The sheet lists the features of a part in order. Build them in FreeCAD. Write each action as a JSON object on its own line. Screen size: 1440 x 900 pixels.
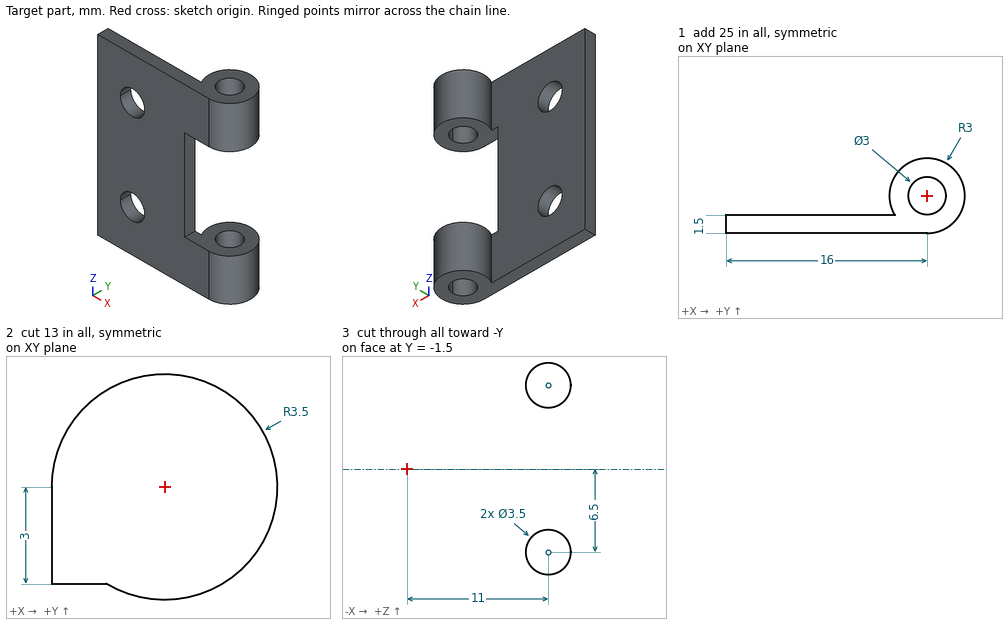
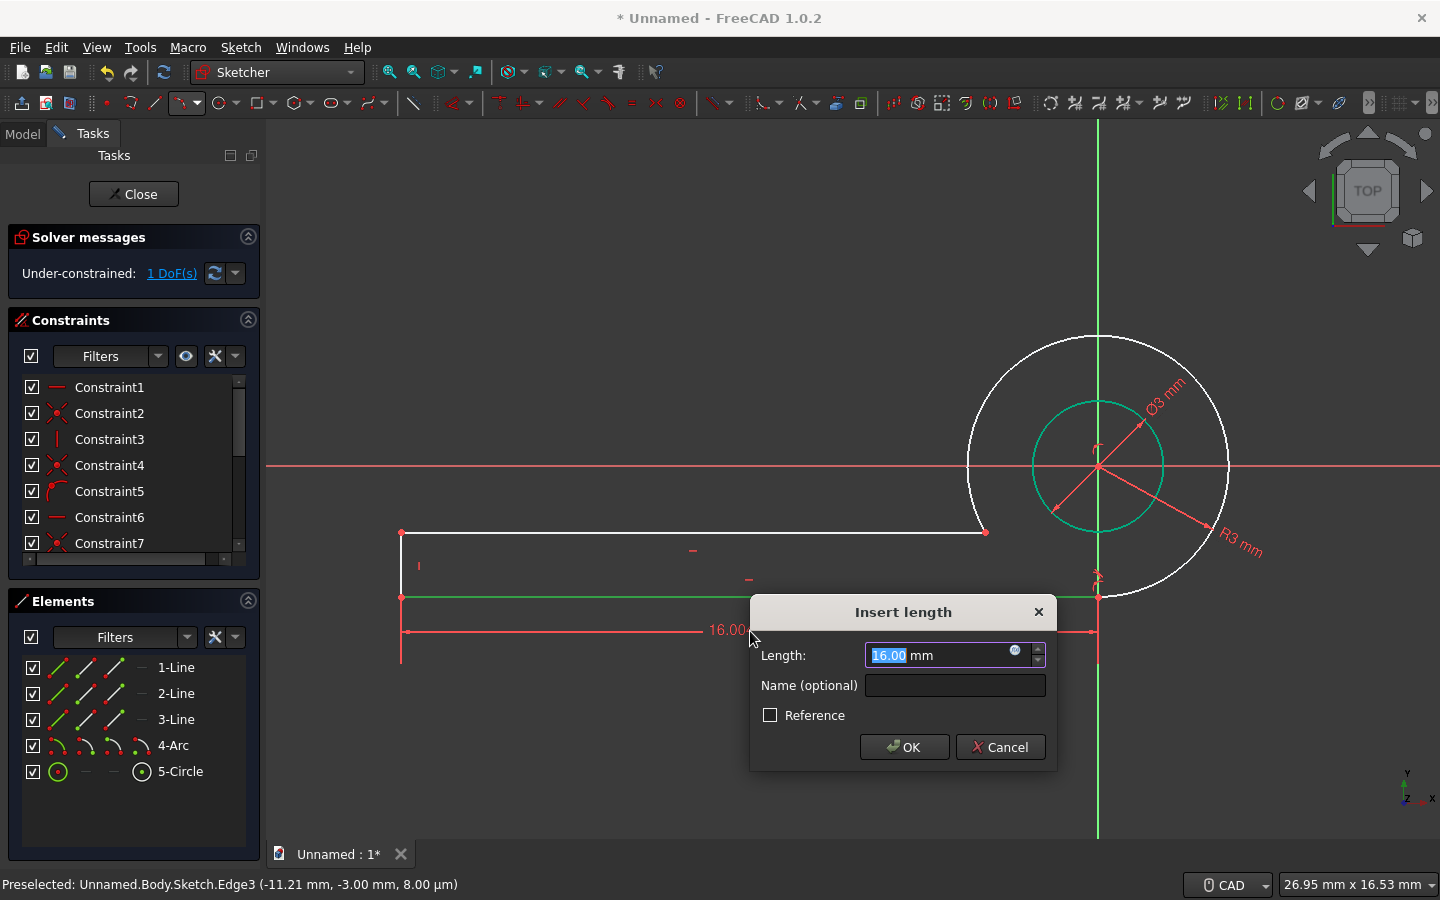
{"action": "type", "text": "16"}
{"action": "key", "text": "Return"}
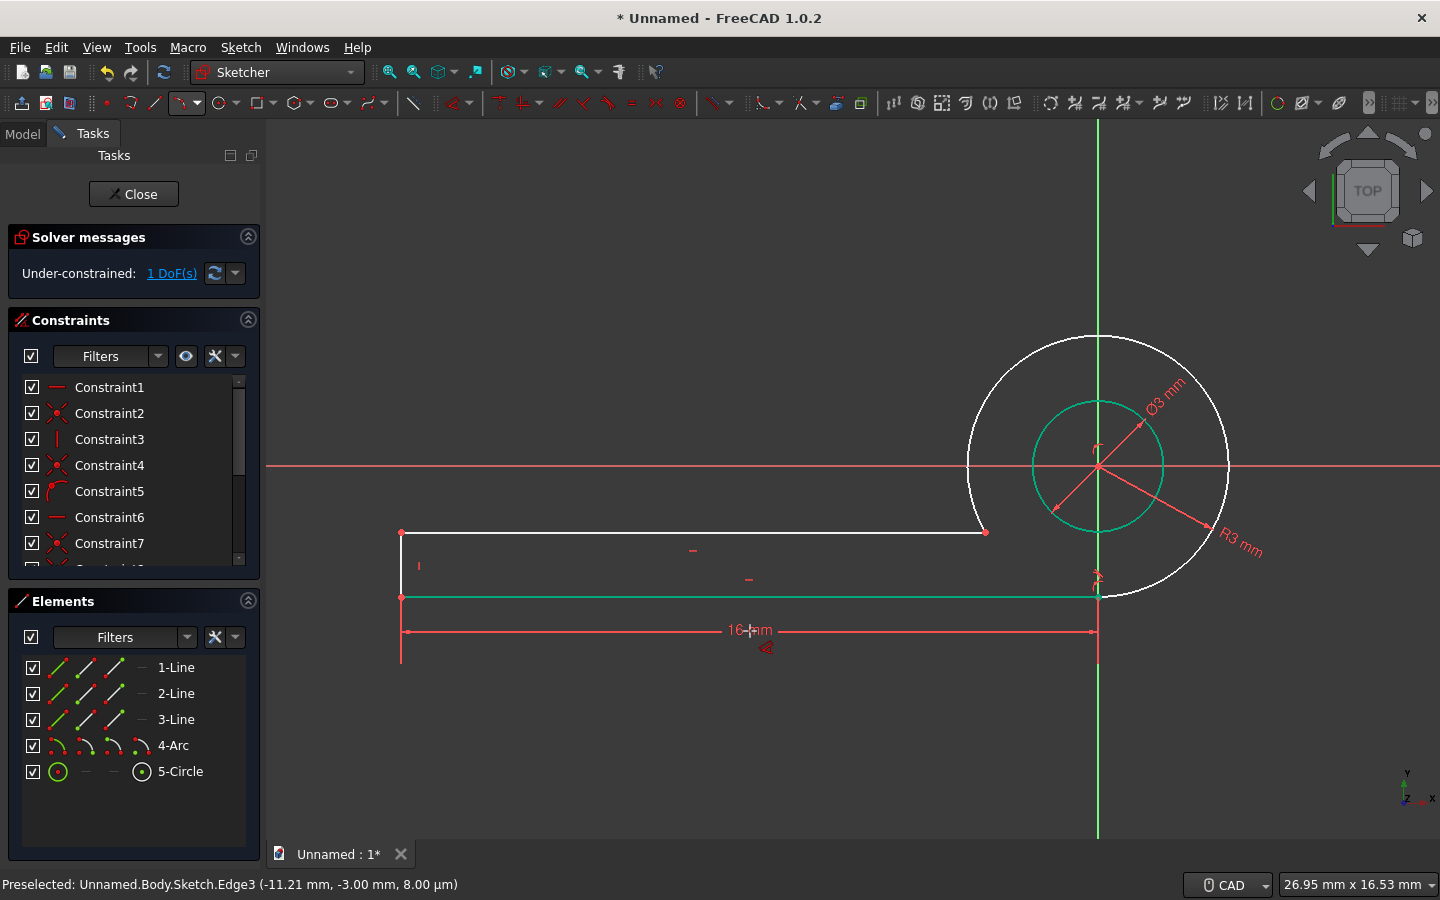
{"action": "left_click", "coordinate": [401, 552]}
{"action": "left_click", "coordinate": [367, 565]}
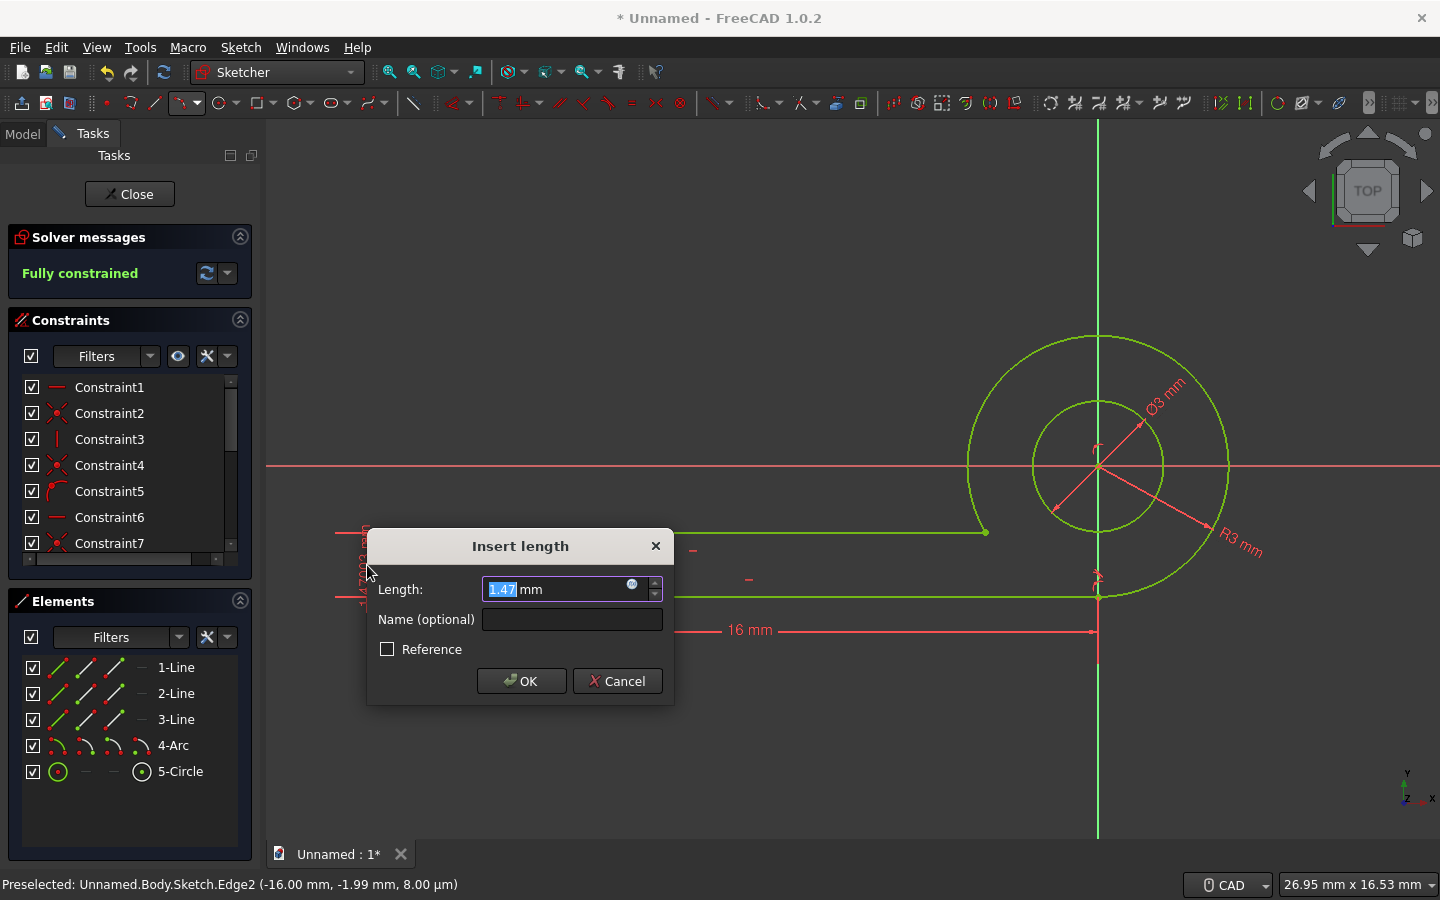
{"action": "type", "text": "1.5"}
{"action": "key", "text": "Return"}
{"action": "key", "text": "Escape"}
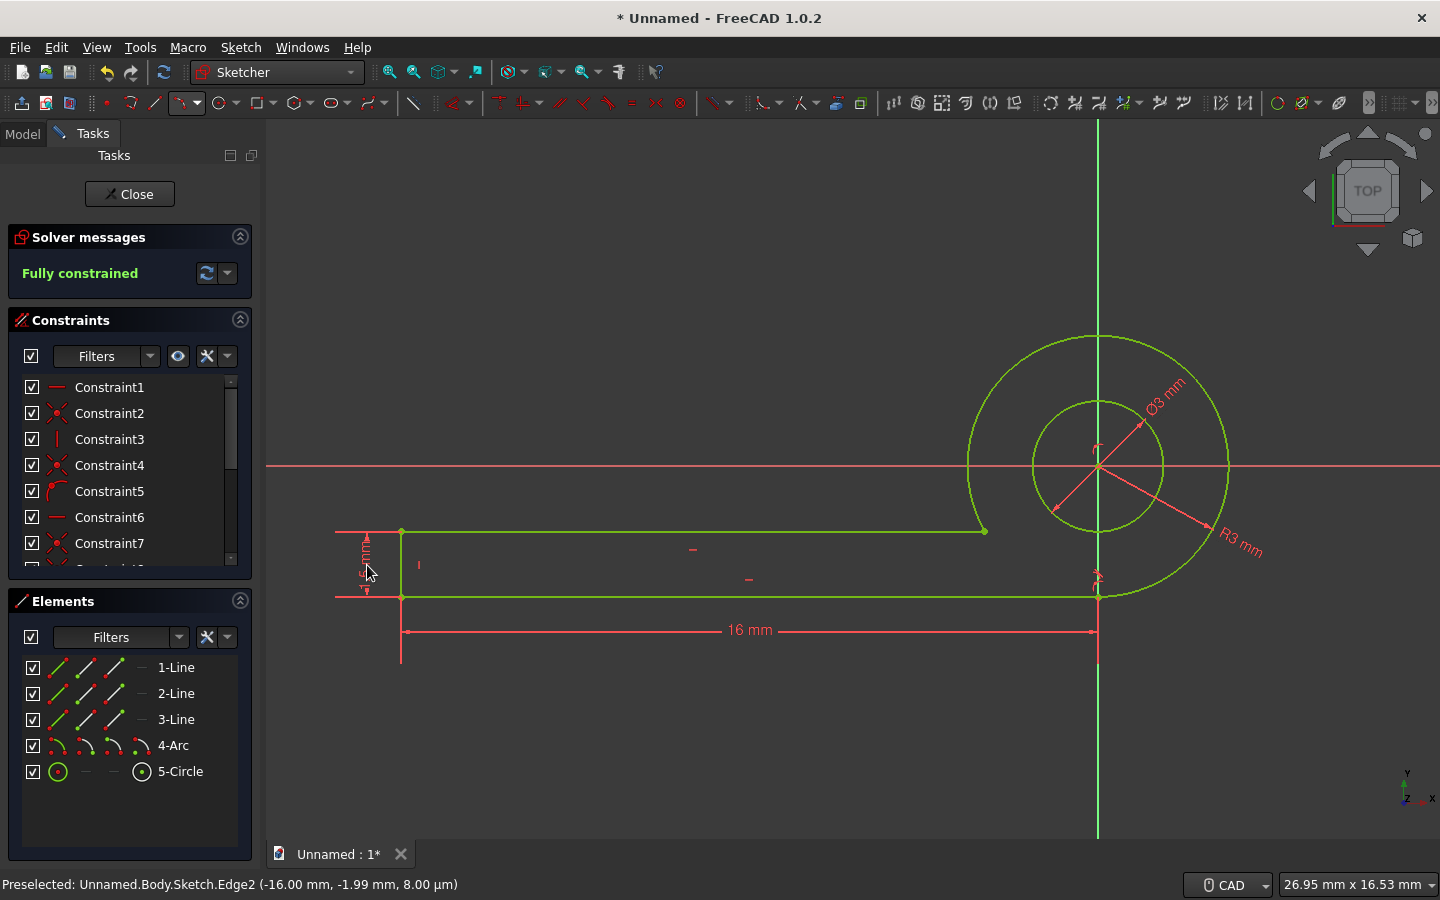
{"action": "left_click", "coordinate": [130, 194]}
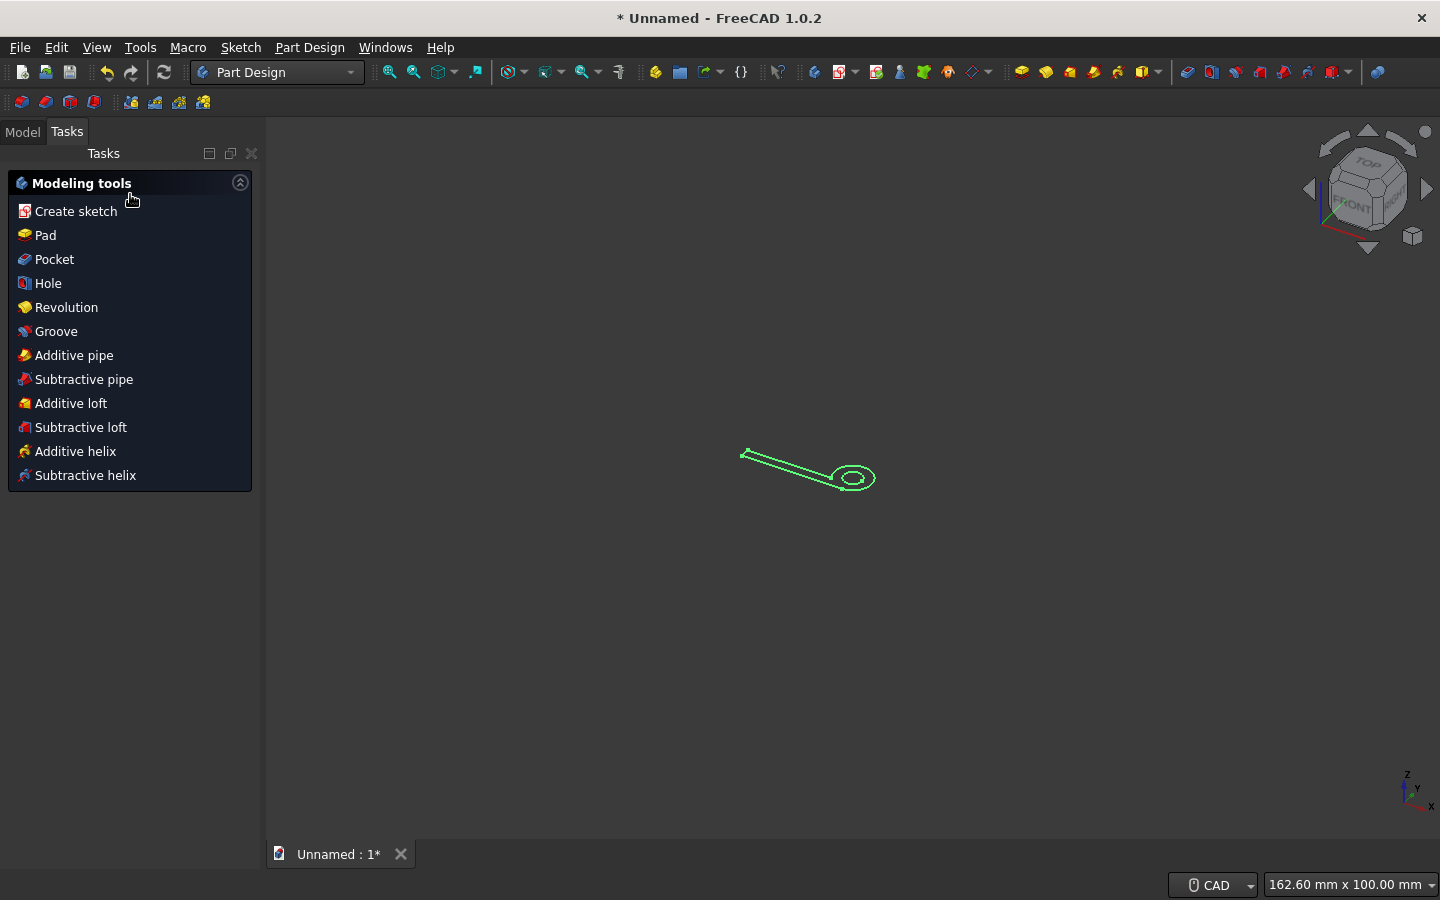
{"action": "left_click", "coordinate": [1022, 72]}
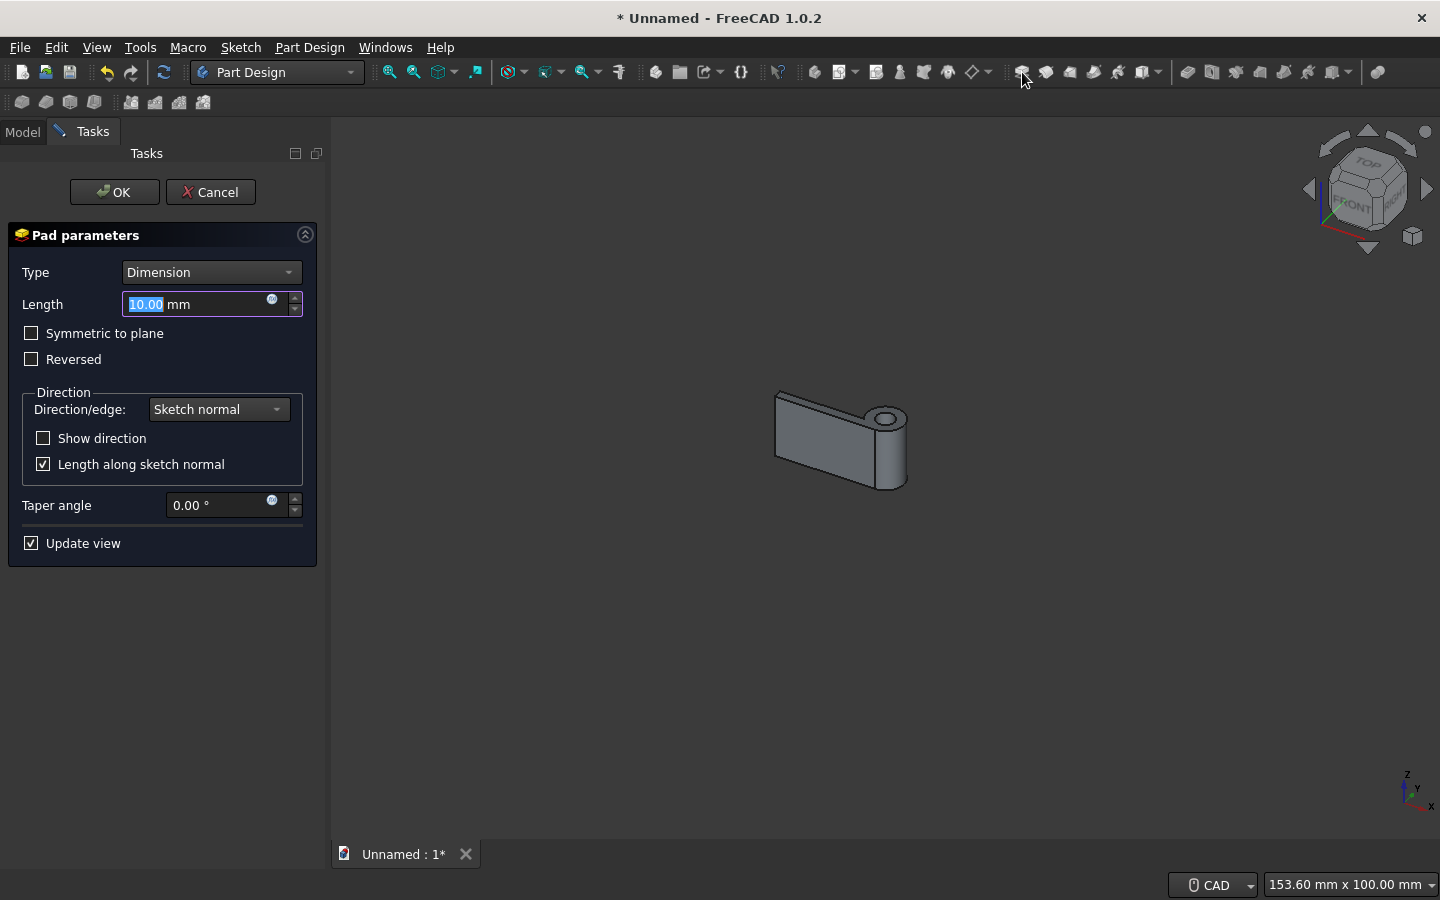
{"action": "type", "text": "25"}
{"action": "key", "text": "Tab"}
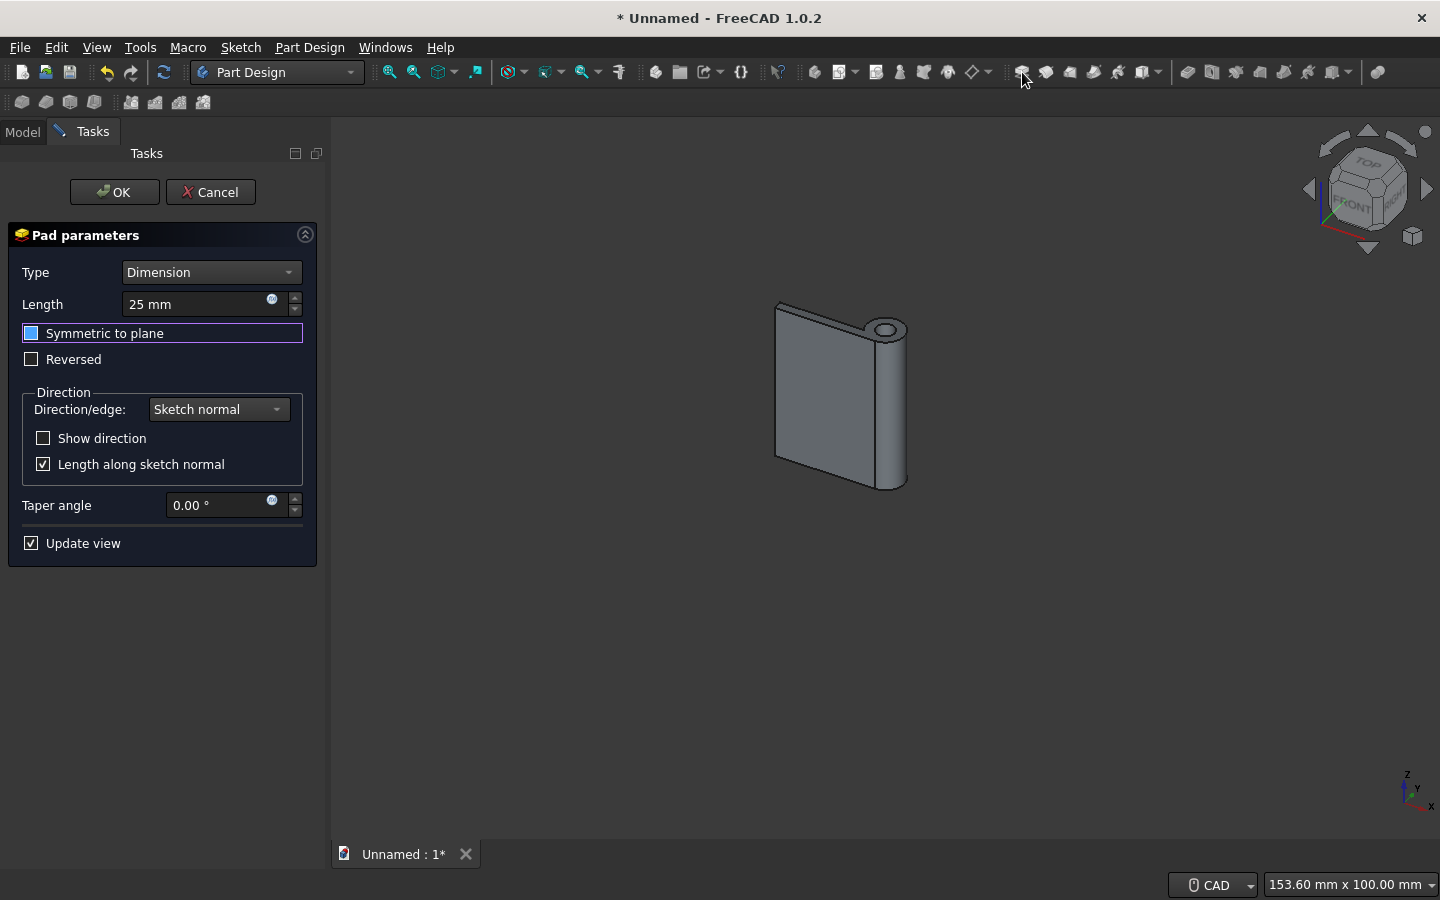
{"action": "left_click", "coordinate": [30, 333]}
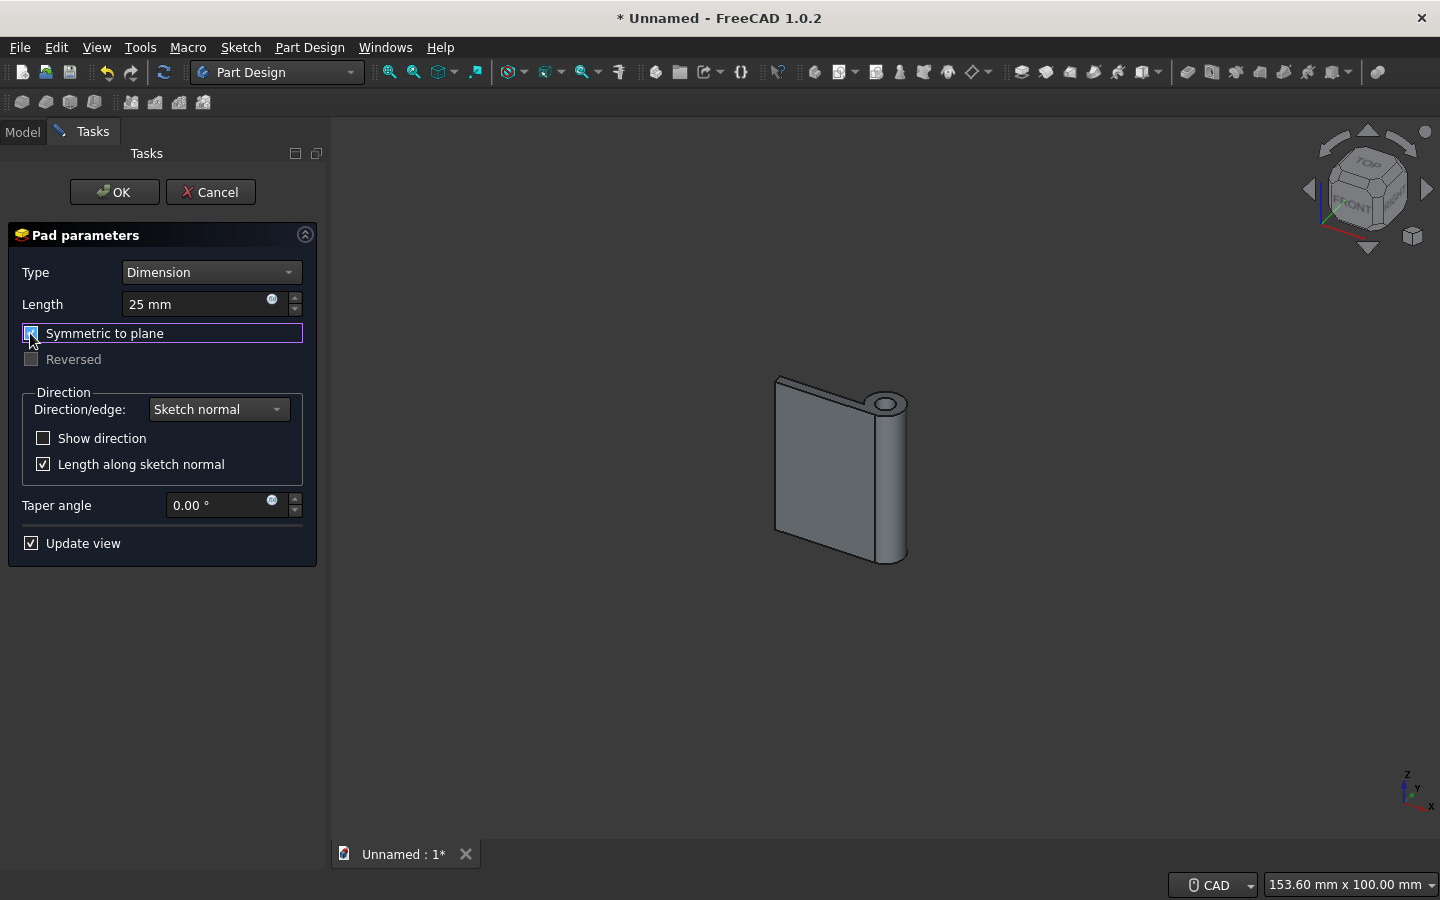
{"action": "left_click", "coordinate": [115, 192]}